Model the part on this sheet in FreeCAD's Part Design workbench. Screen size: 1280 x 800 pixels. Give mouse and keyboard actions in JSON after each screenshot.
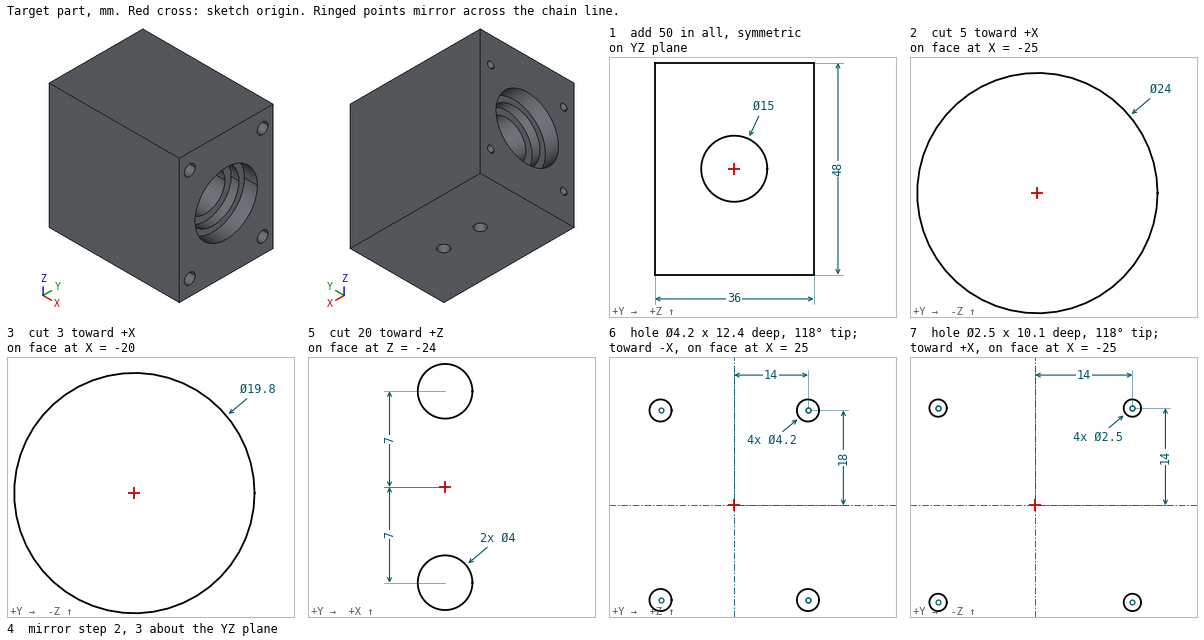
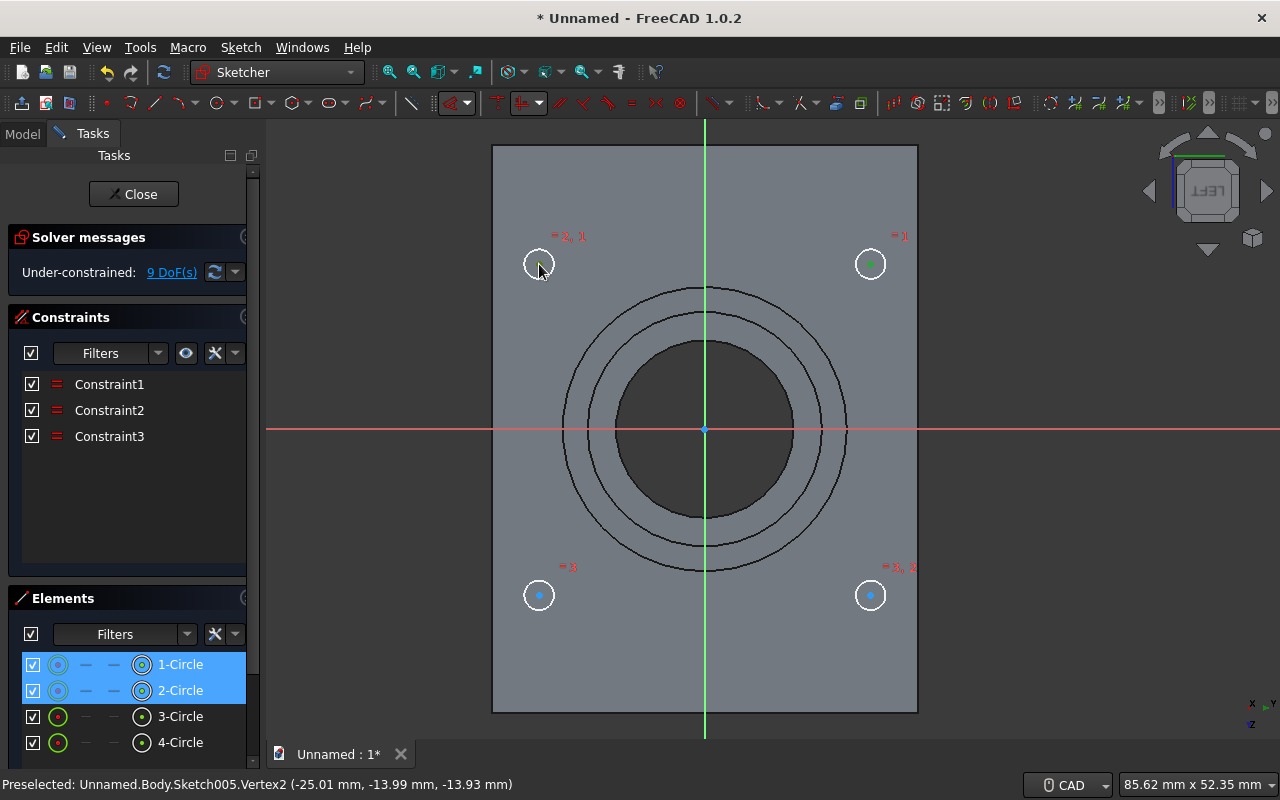
{"action": "left_click", "coordinate": [705, 671]}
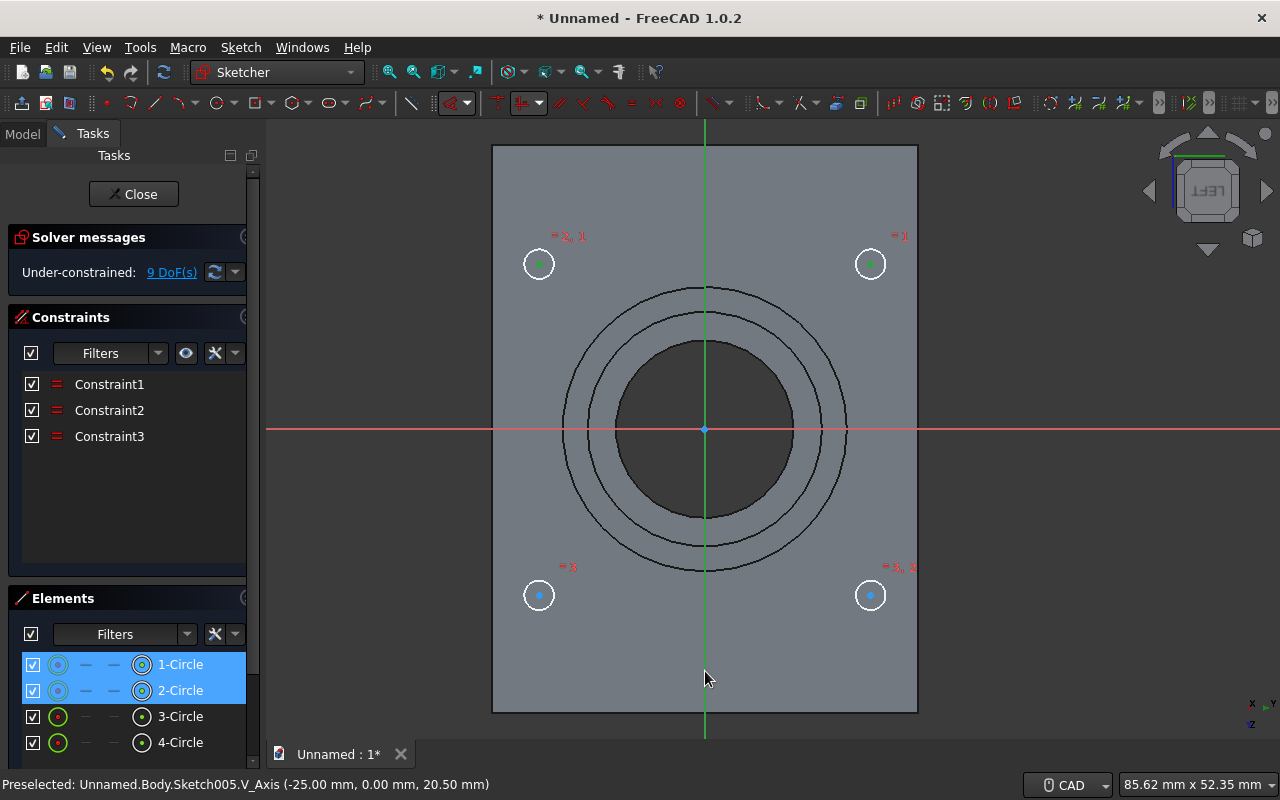
{"action": "left_click", "coordinate": [656, 104]}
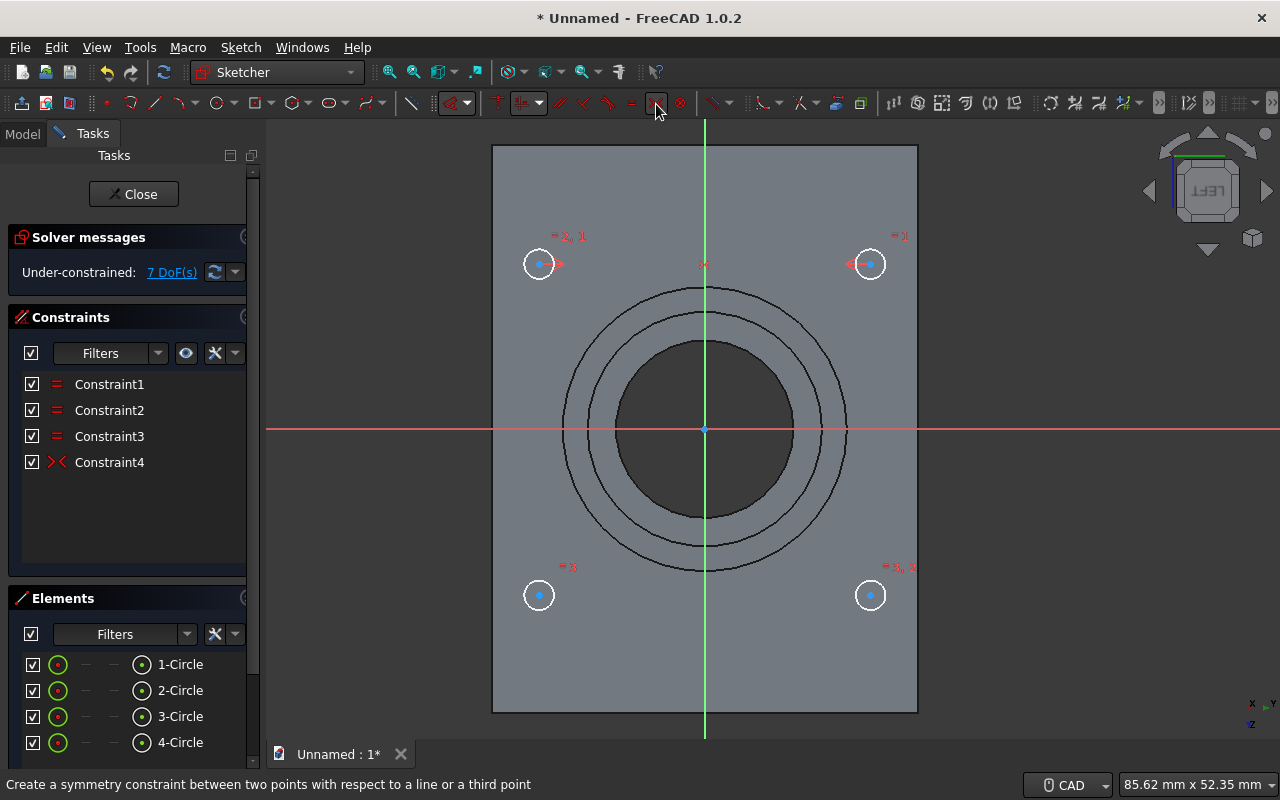
{"action": "left_click", "coordinate": [870, 264]}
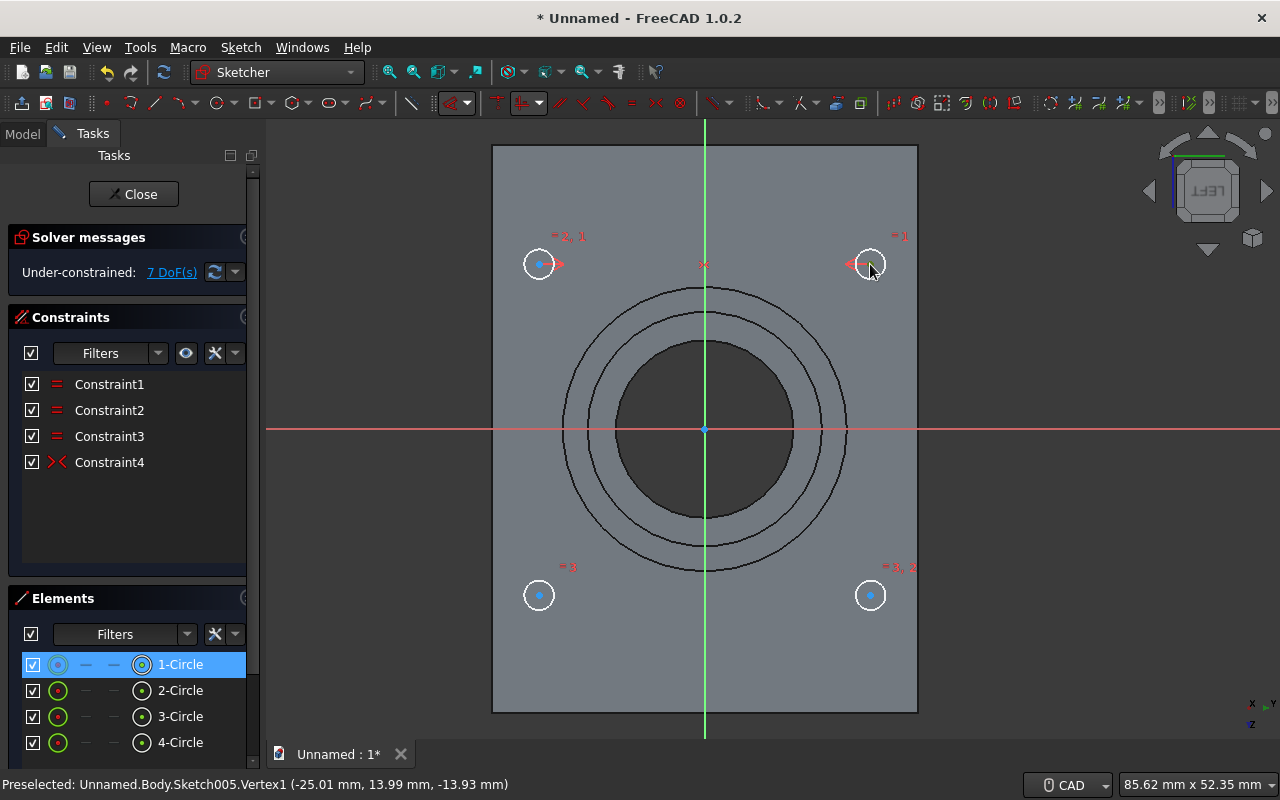
{"action": "left_click", "coordinate": [871, 595]}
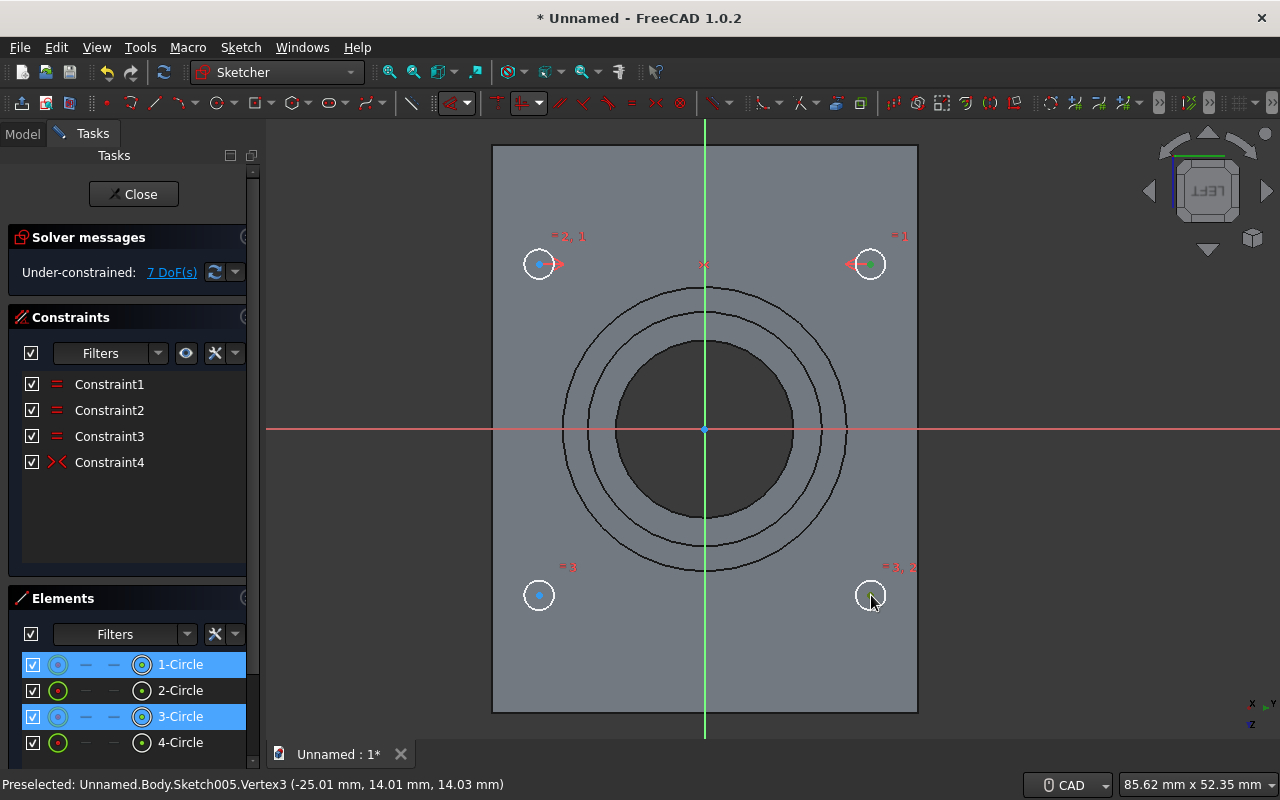
{"action": "left_click", "coordinate": [353, 429]}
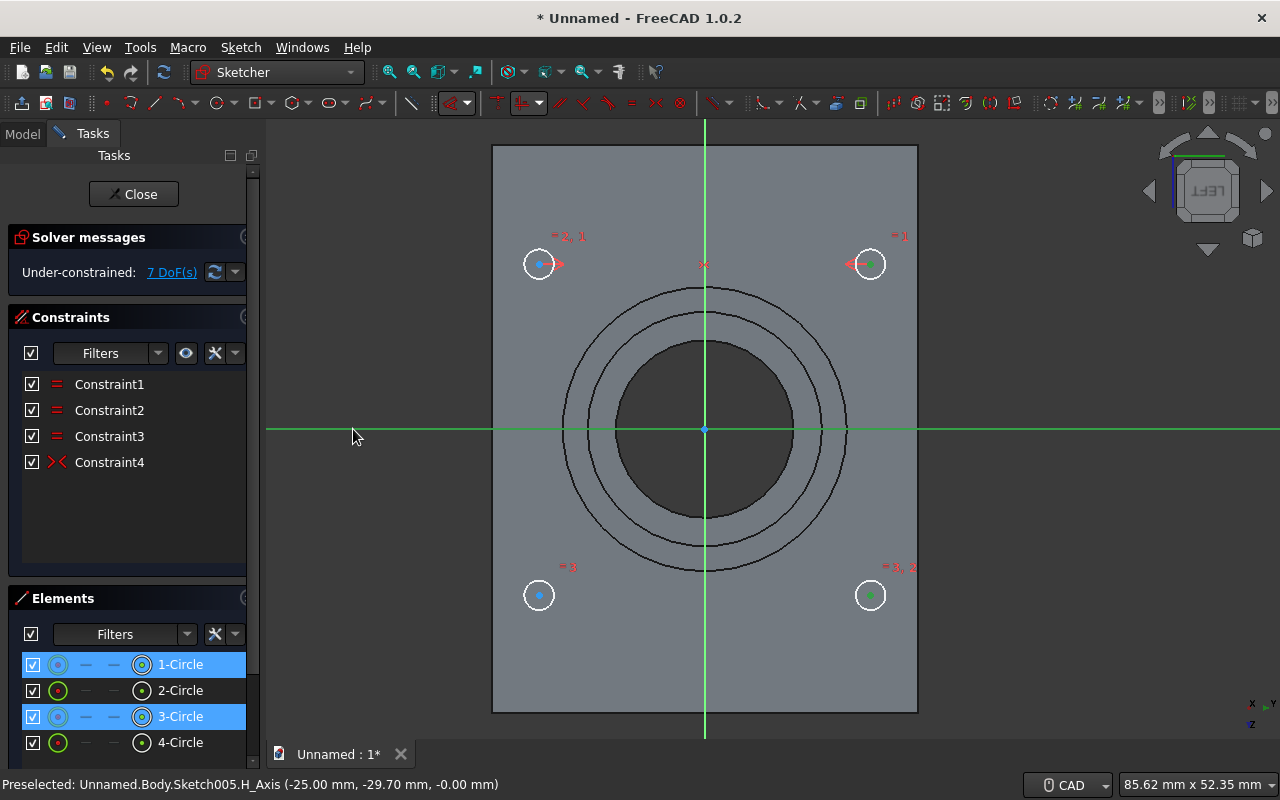
{"action": "left_click", "coordinate": [656, 104]}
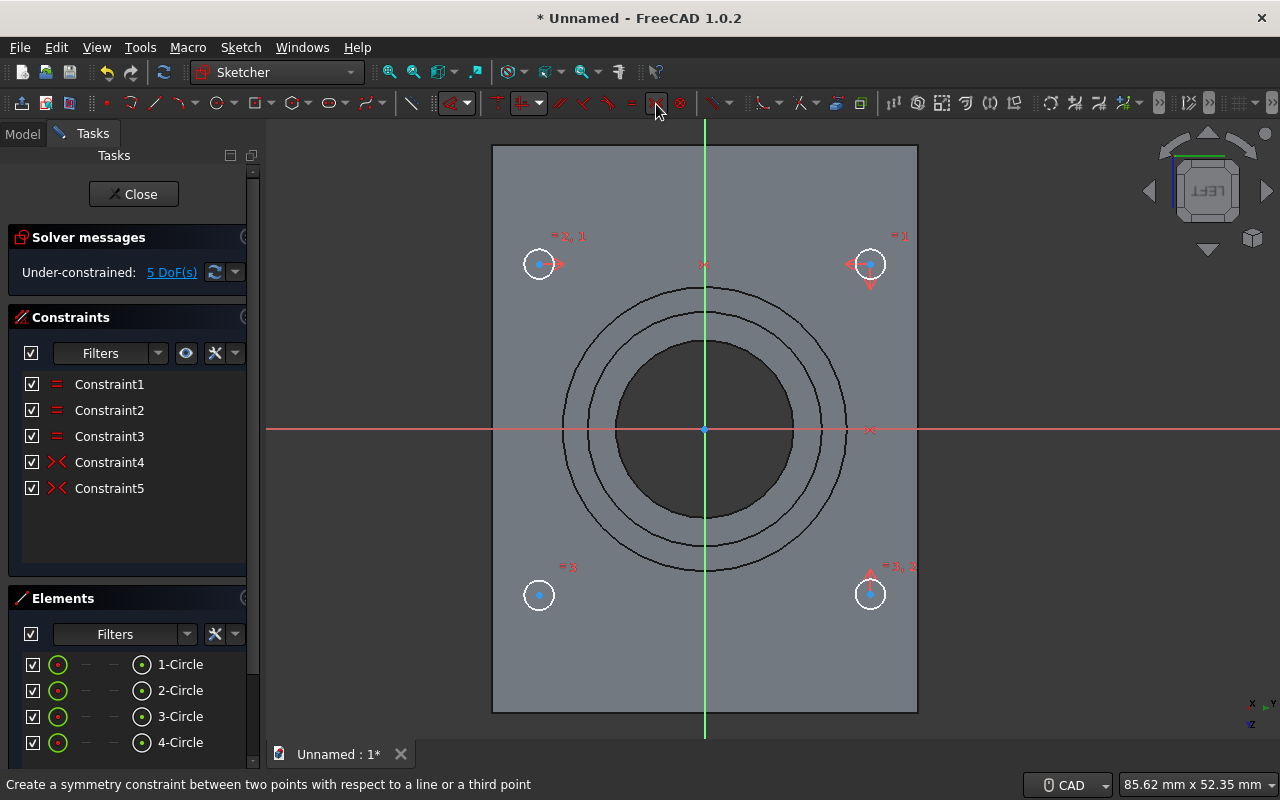
{"action": "left_click", "coordinate": [539, 264]}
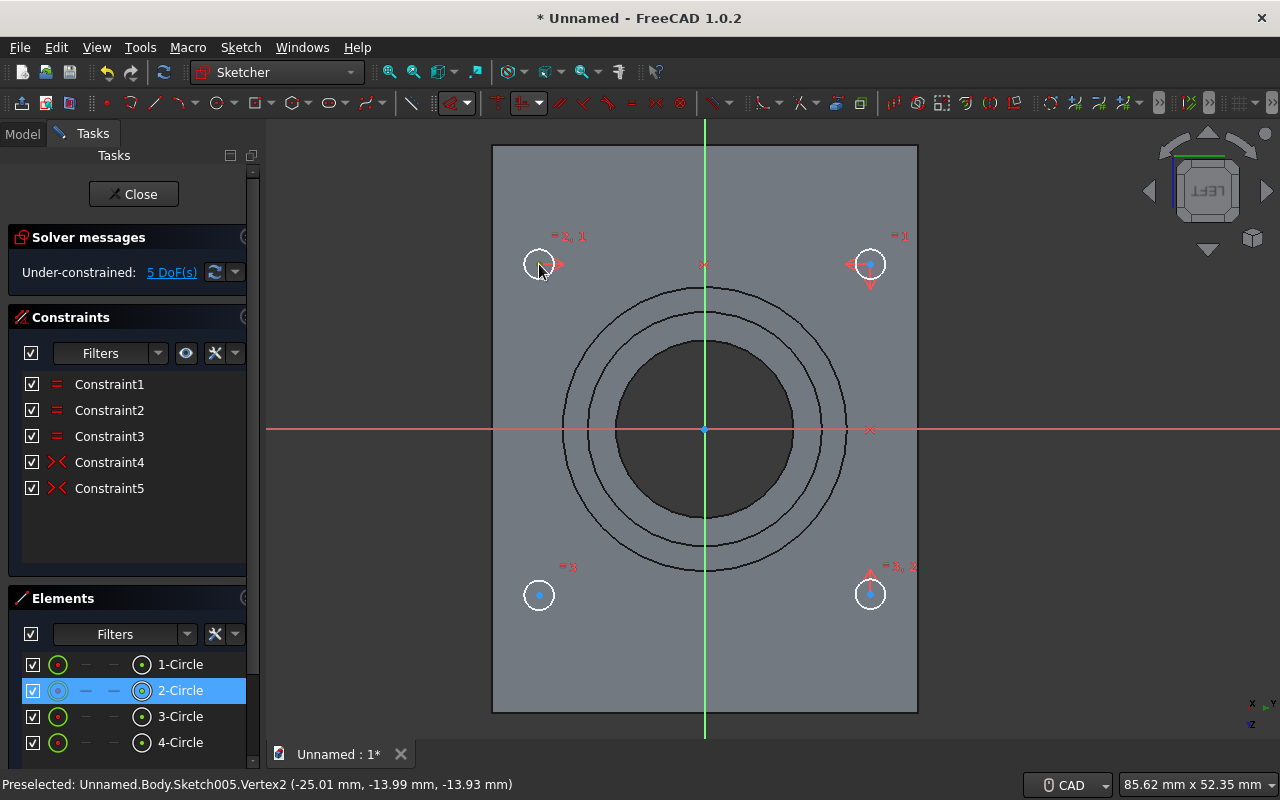
{"action": "left_click", "coordinate": [539, 595]}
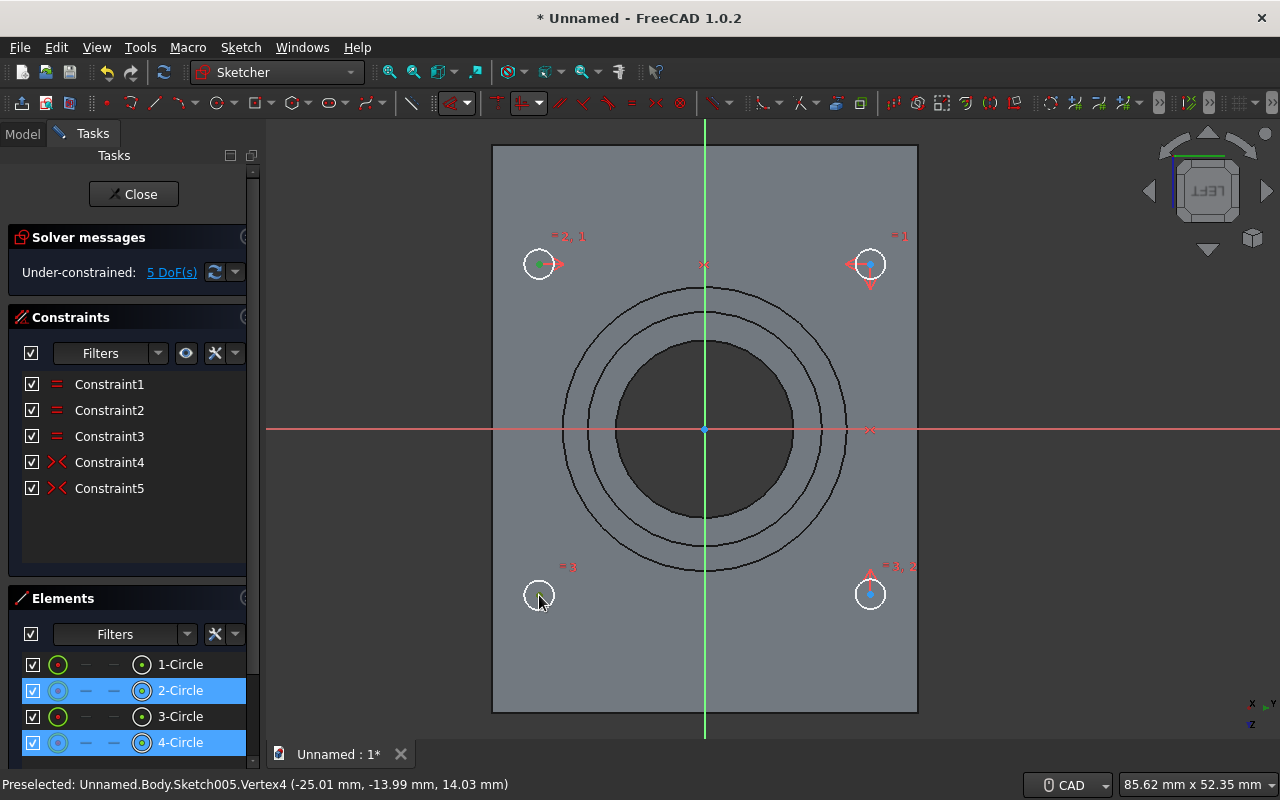
{"action": "left_click", "coordinate": [353, 429]}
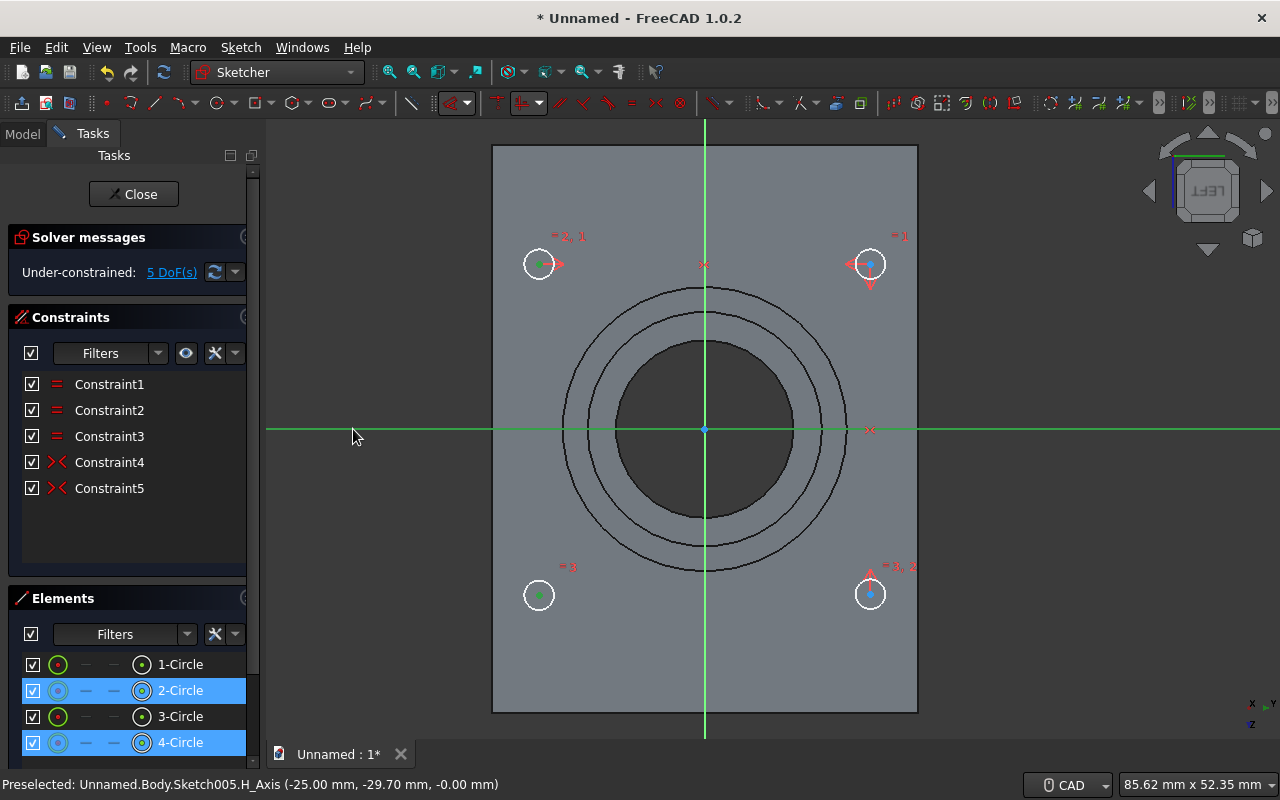
{"action": "left_click", "coordinate": [656, 104]}